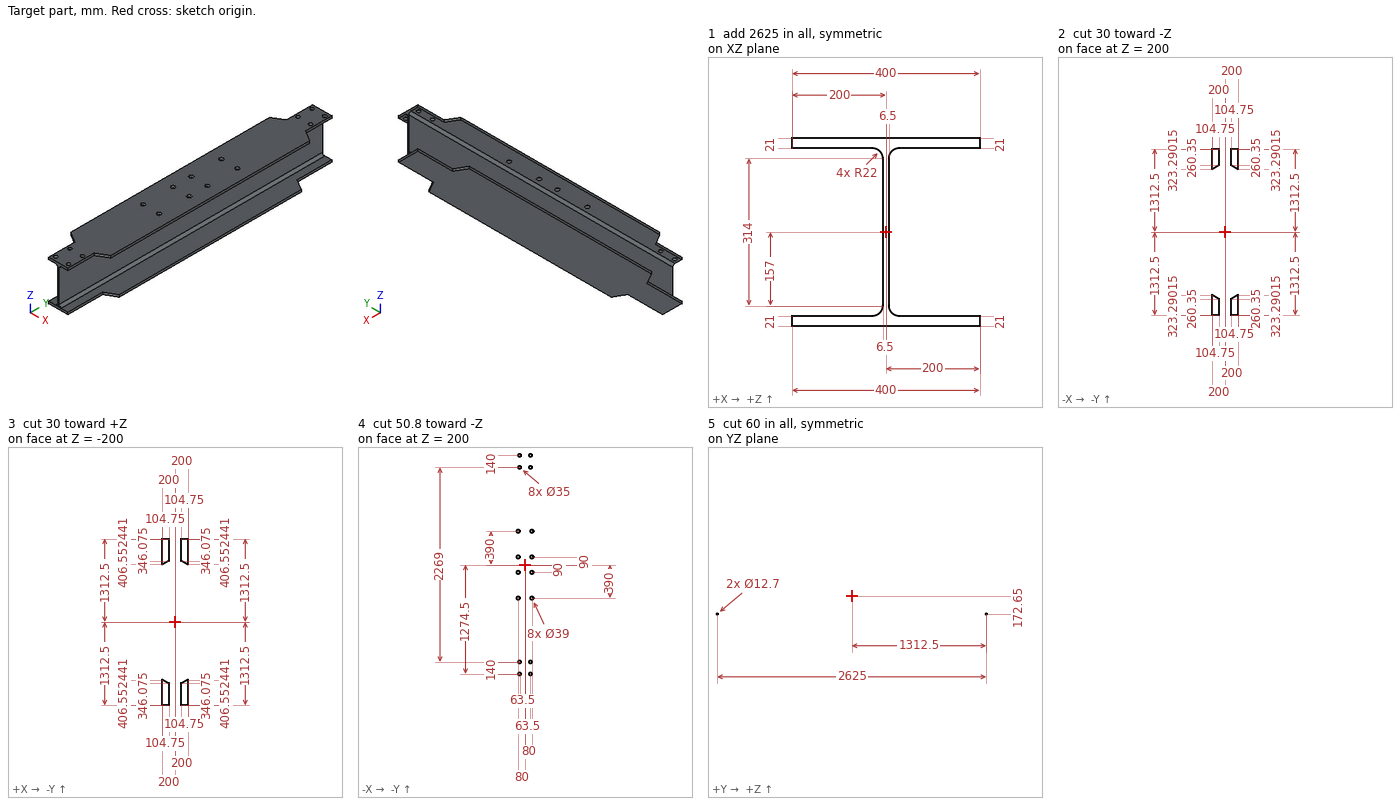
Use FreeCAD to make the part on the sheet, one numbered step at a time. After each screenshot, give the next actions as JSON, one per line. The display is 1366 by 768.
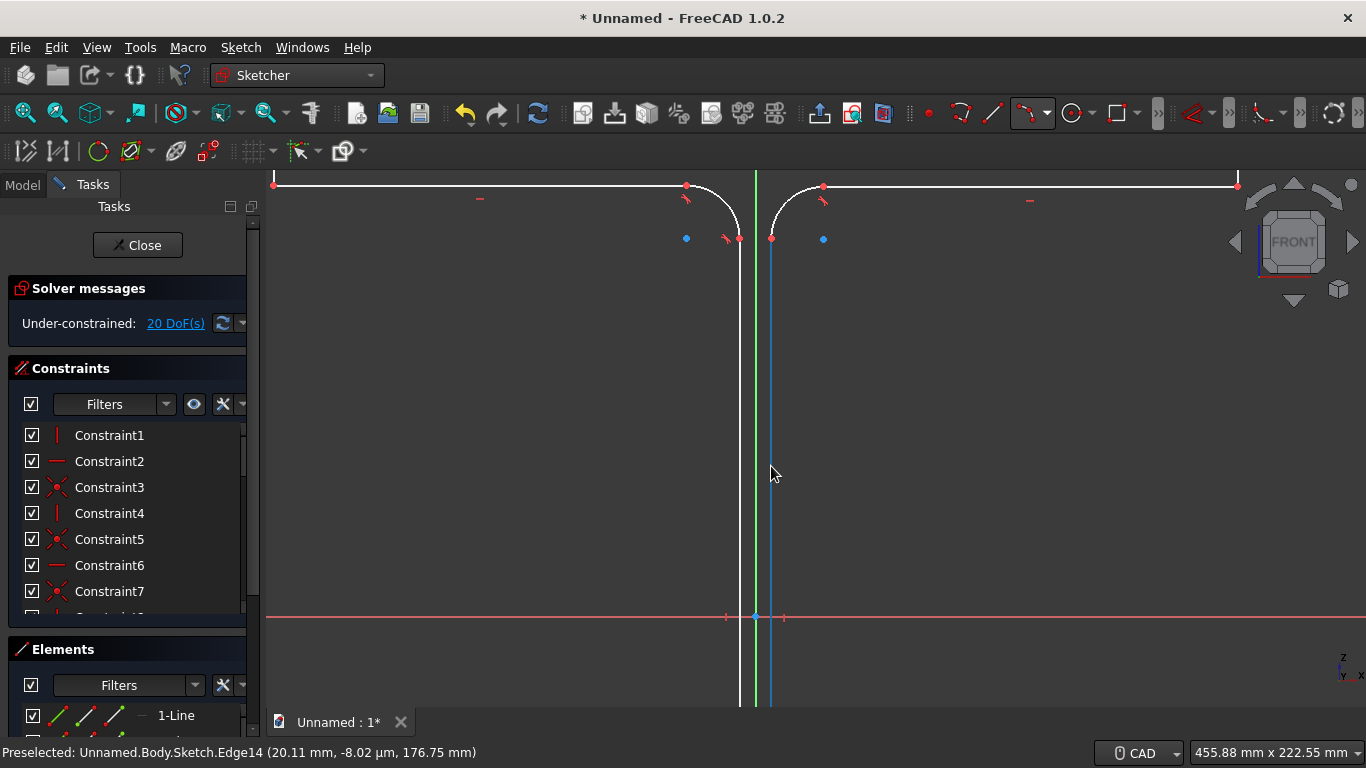
{"action": "left_click", "coordinate": [771, 466]}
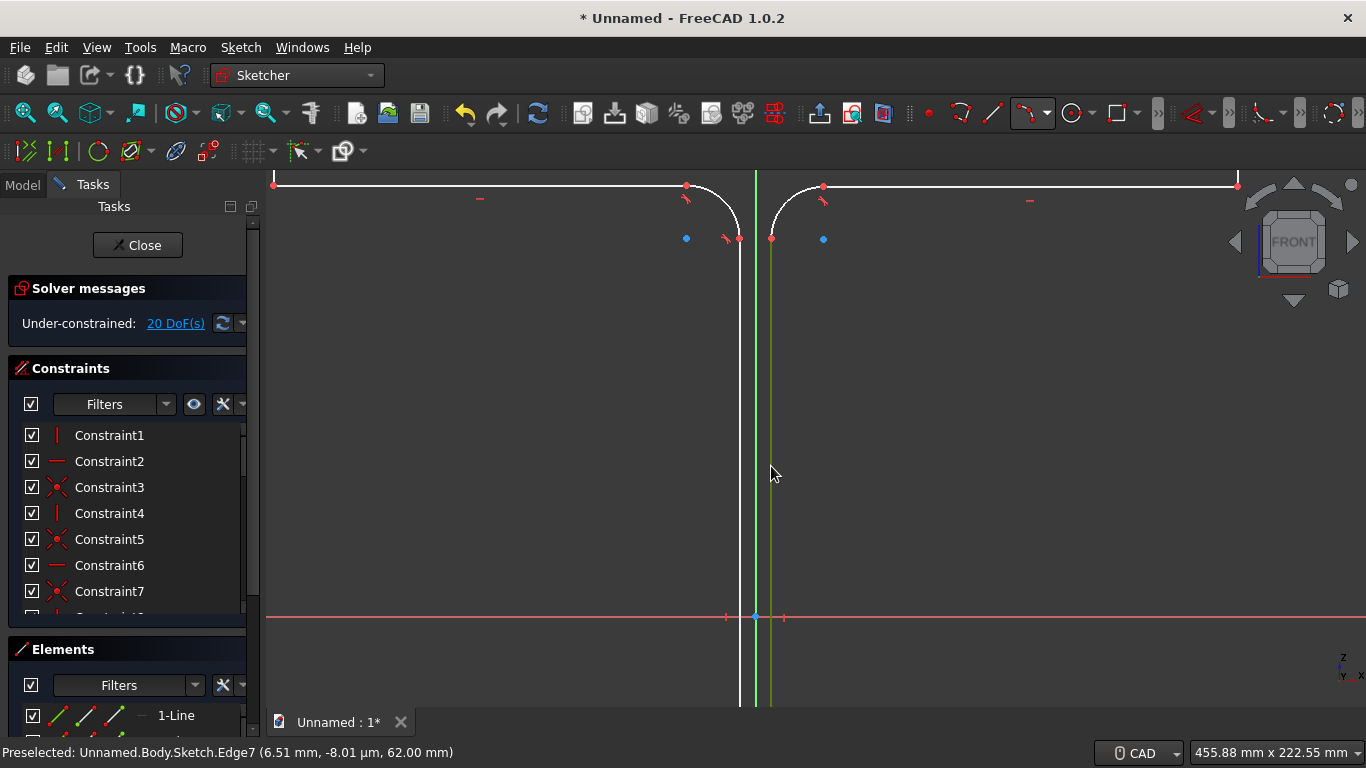
{"action": "left_click", "coordinate": [777, 215]}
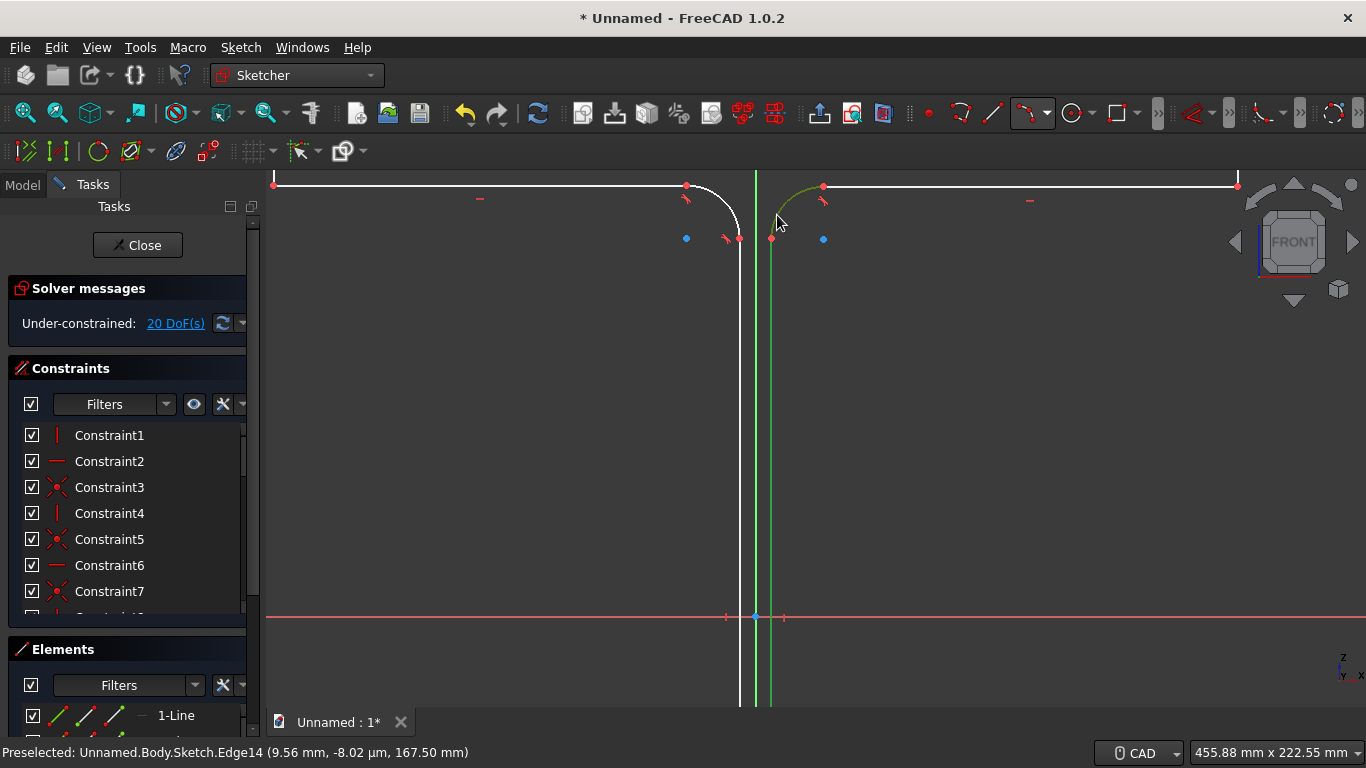
{"action": "key", "text": "t"}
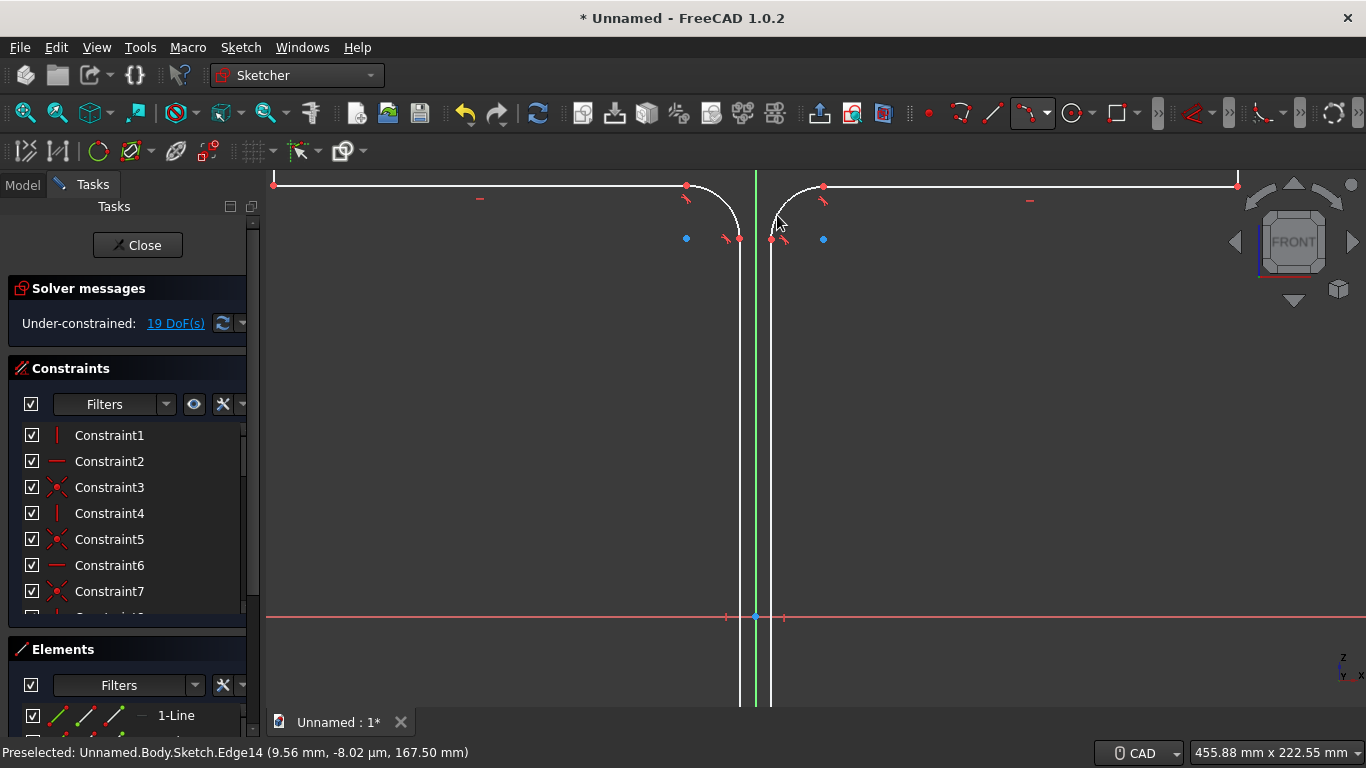
{"action": "left_click", "coordinate": [771, 466]}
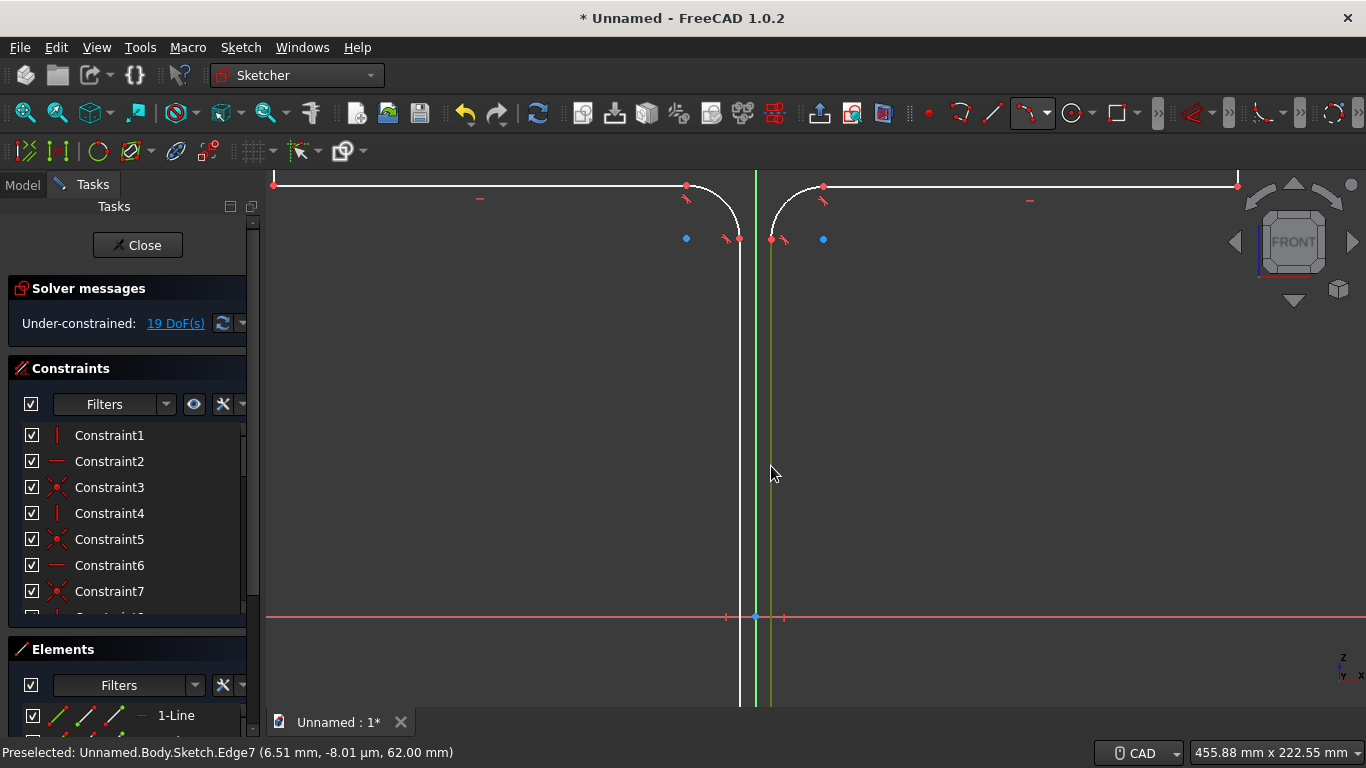
{"action": "scroll", "coordinate": [743, 335], "scroll_direction": "down", "scroll_amount": 5}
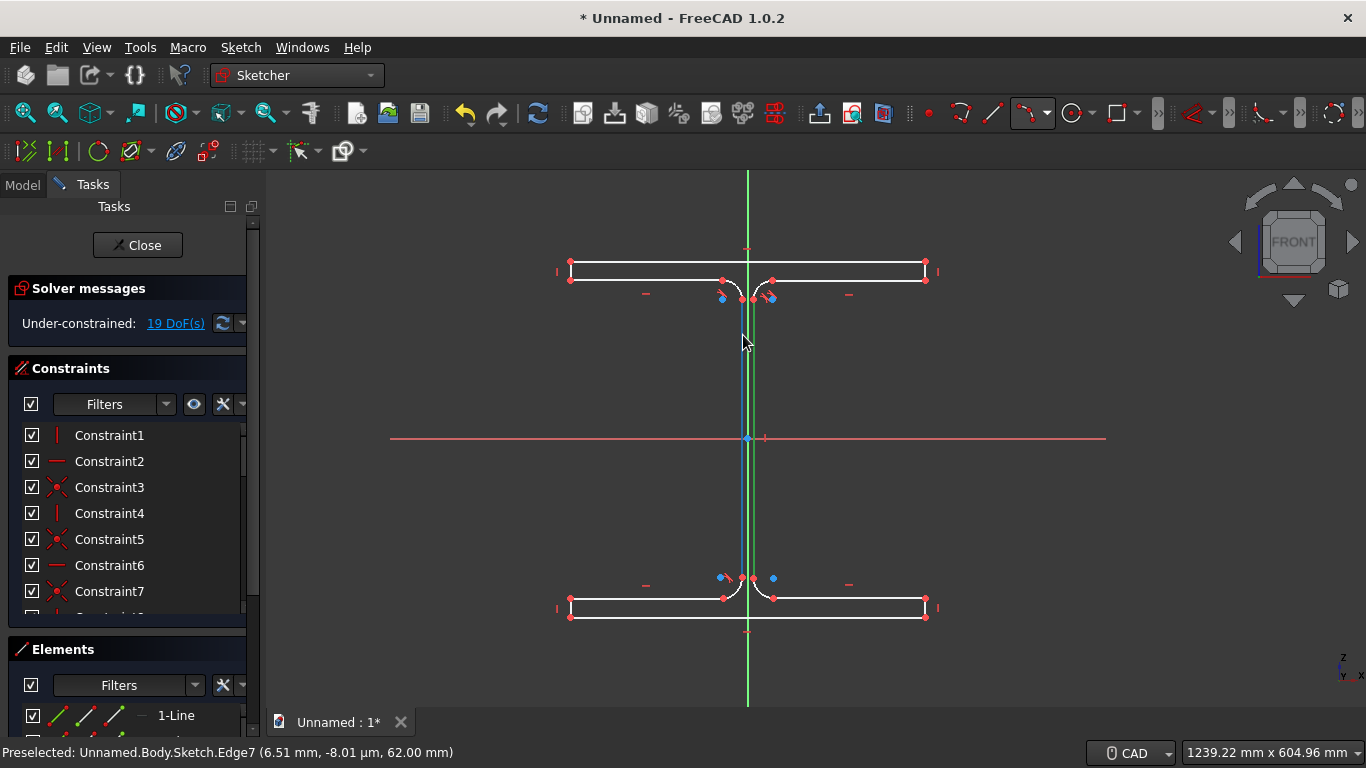
{"action": "scroll", "coordinate": [756, 587], "scroll_direction": "up", "scroll_amount": 3}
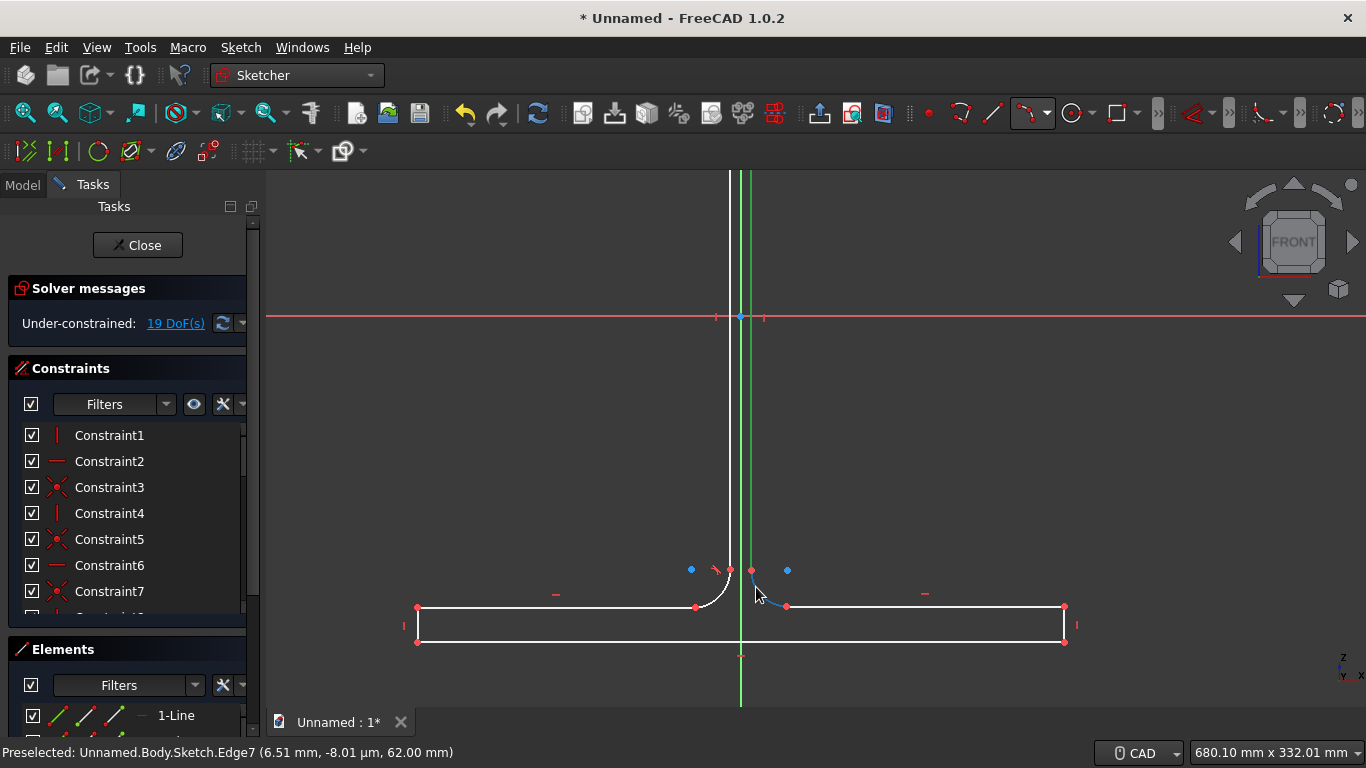
{"action": "left_click", "coordinate": [755, 587]}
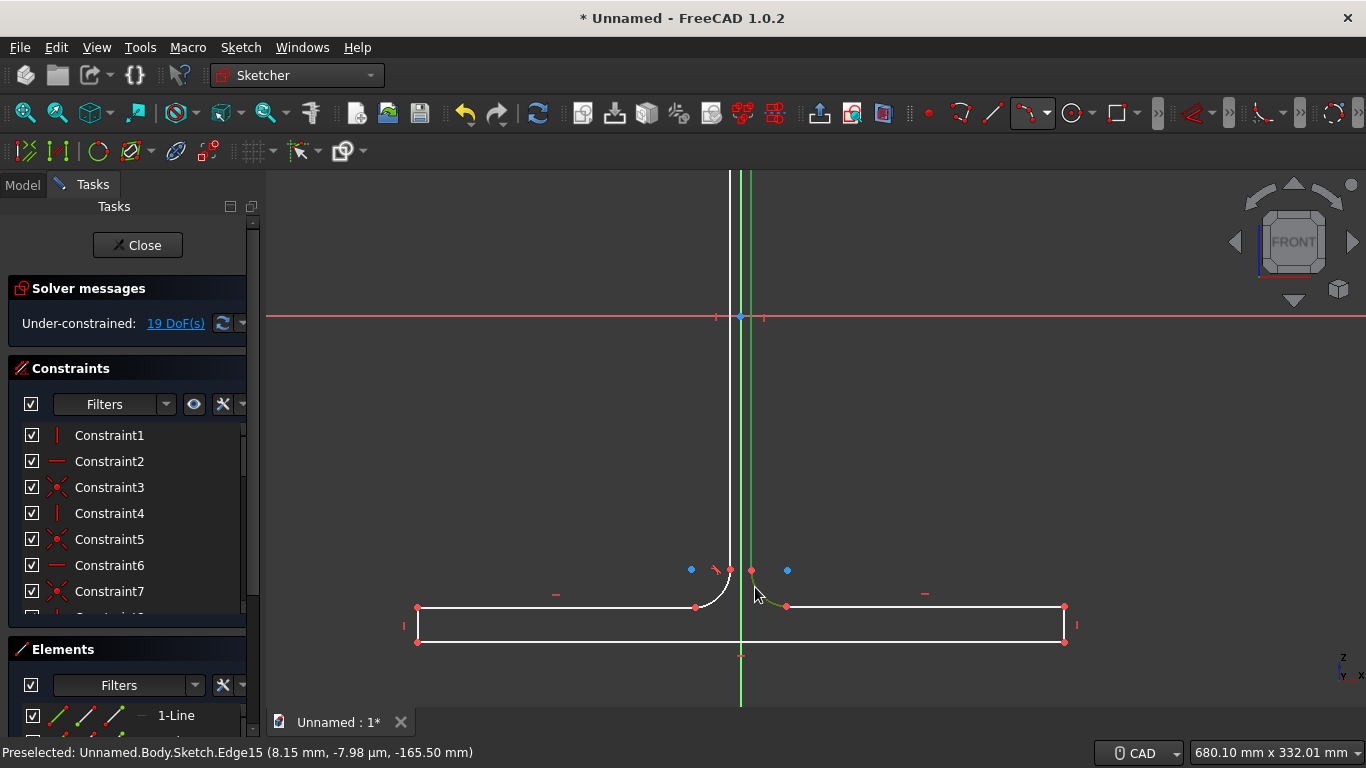
{"action": "key", "text": "t"}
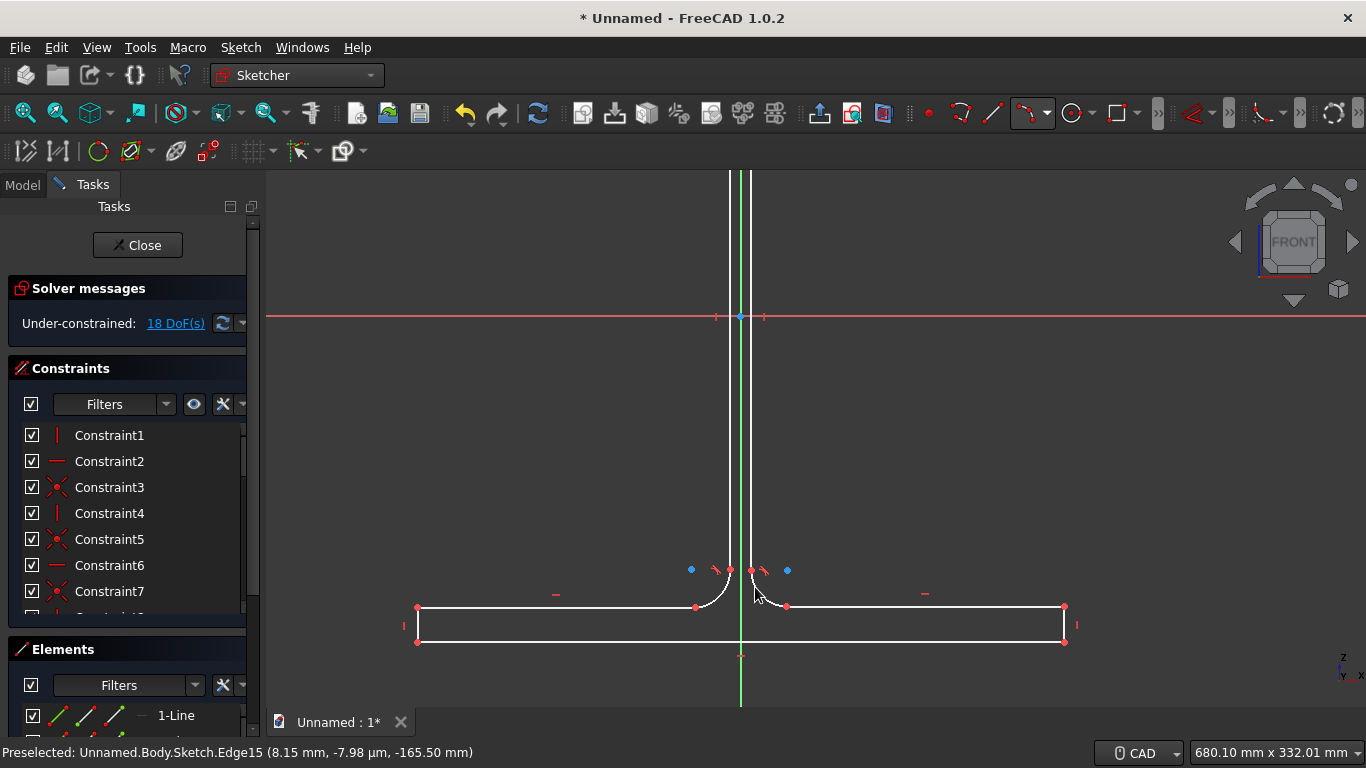
{"action": "left_click", "coordinate": [870, 607]}